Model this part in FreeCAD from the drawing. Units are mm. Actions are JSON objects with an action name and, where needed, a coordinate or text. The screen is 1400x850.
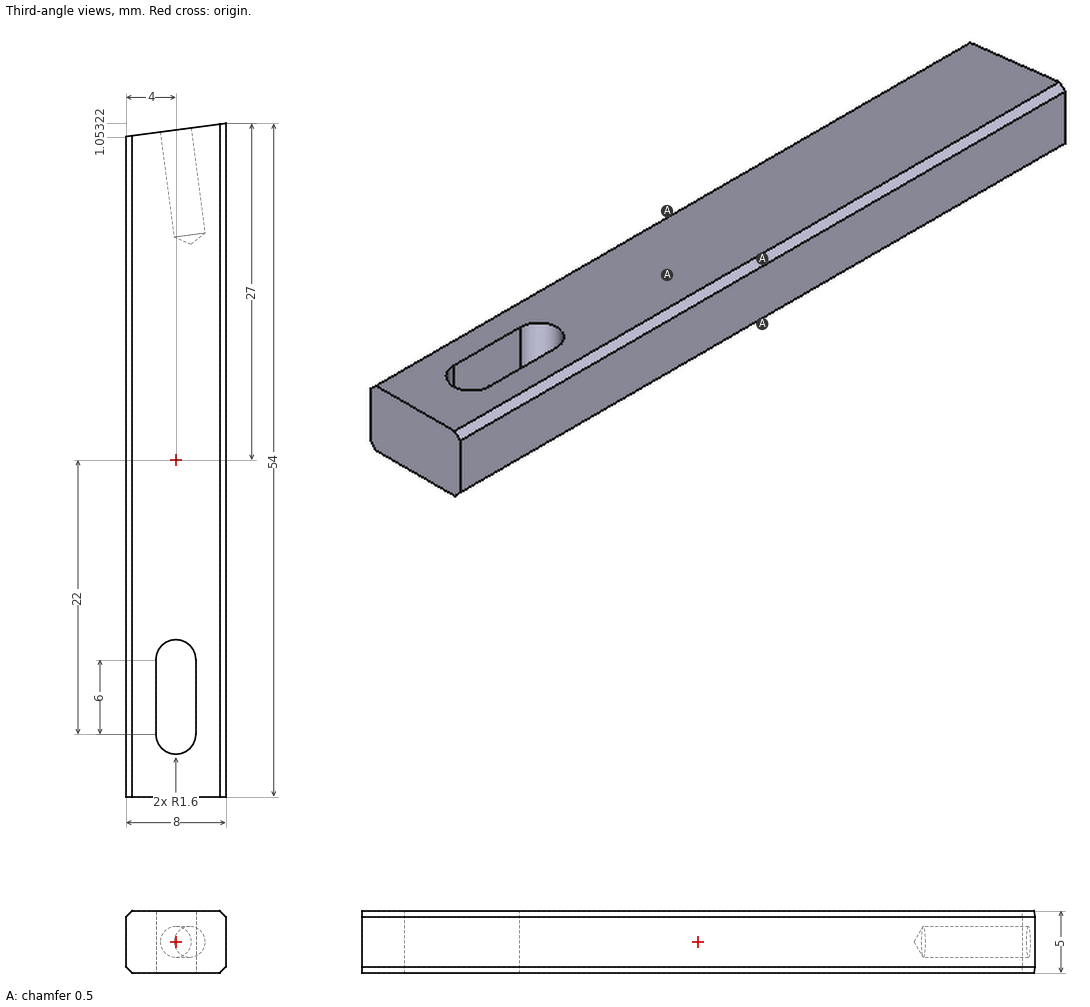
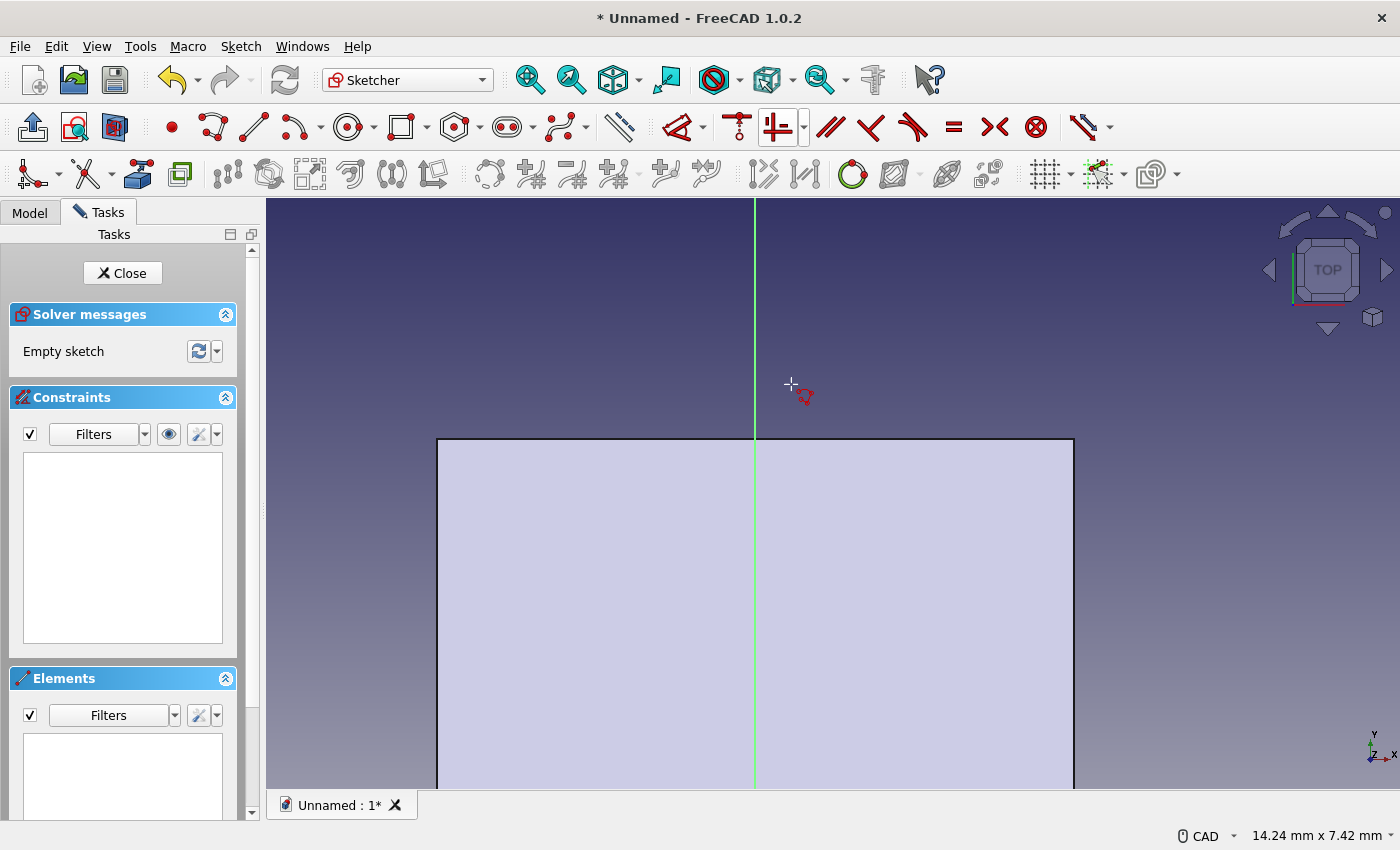
{"action": "left_click", "coordinate": [437, 523]}
{"action": "left_click", "coordinate": [1074, 439]}
{"action": "left_click", "coordinate": [437, 439]}
{"action": "left_click", "coordinate": [437, 524]}
{"action": "key", "text": "Escape"}
{"action": "key", "text": "Escape"}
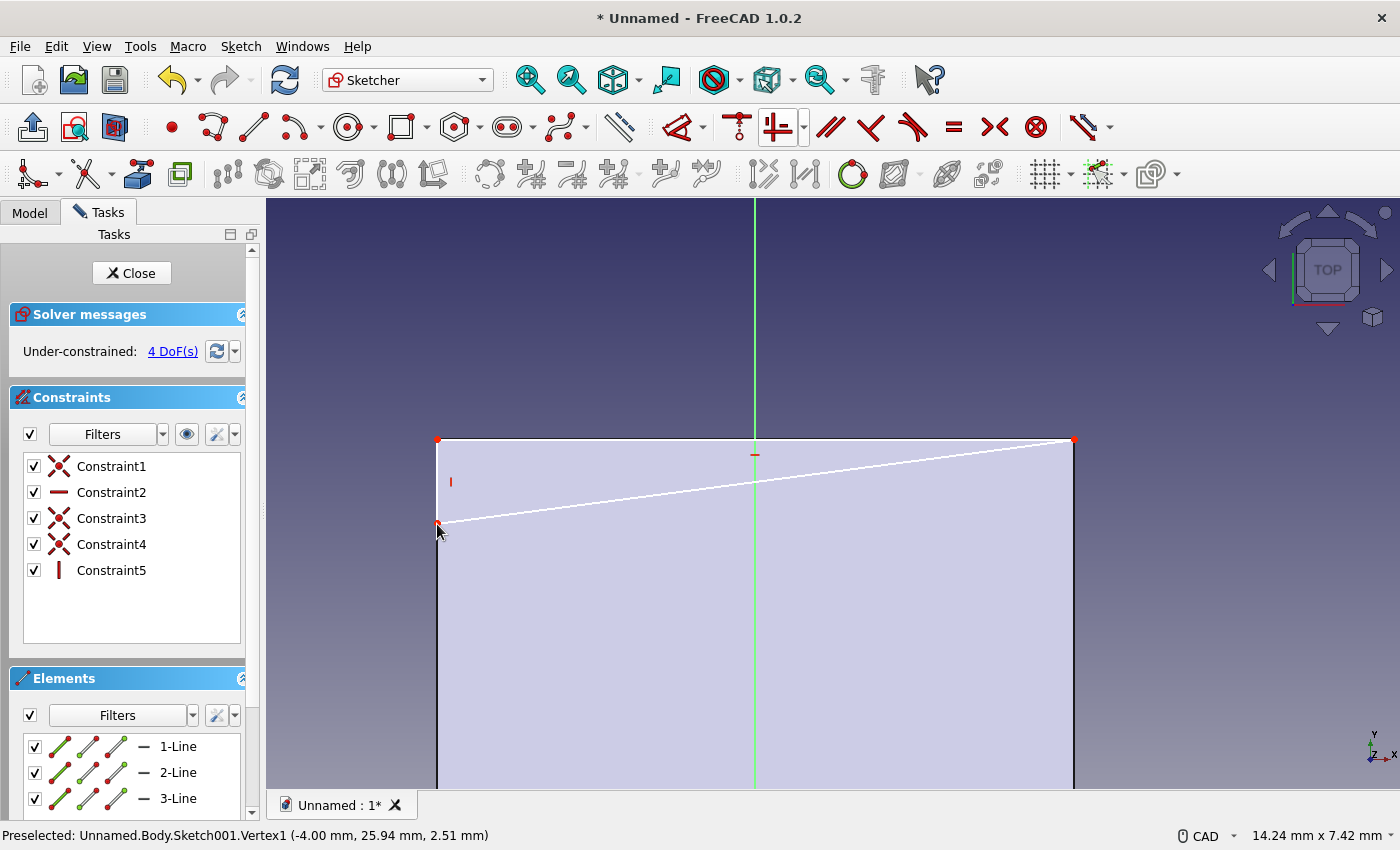
{"action": "left_click", "coordinate": [883, 440]}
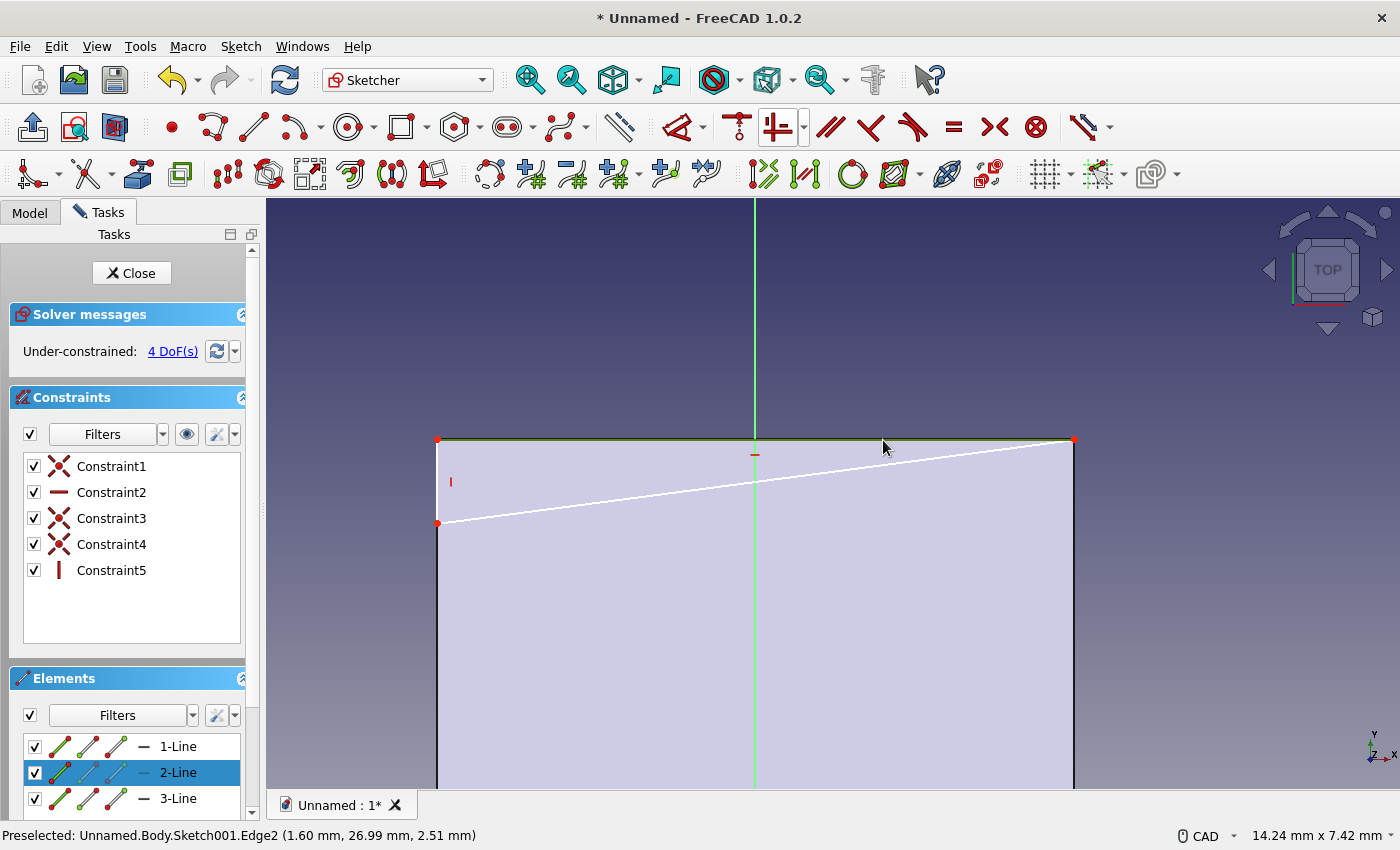
{"action": "key", "text": "l"}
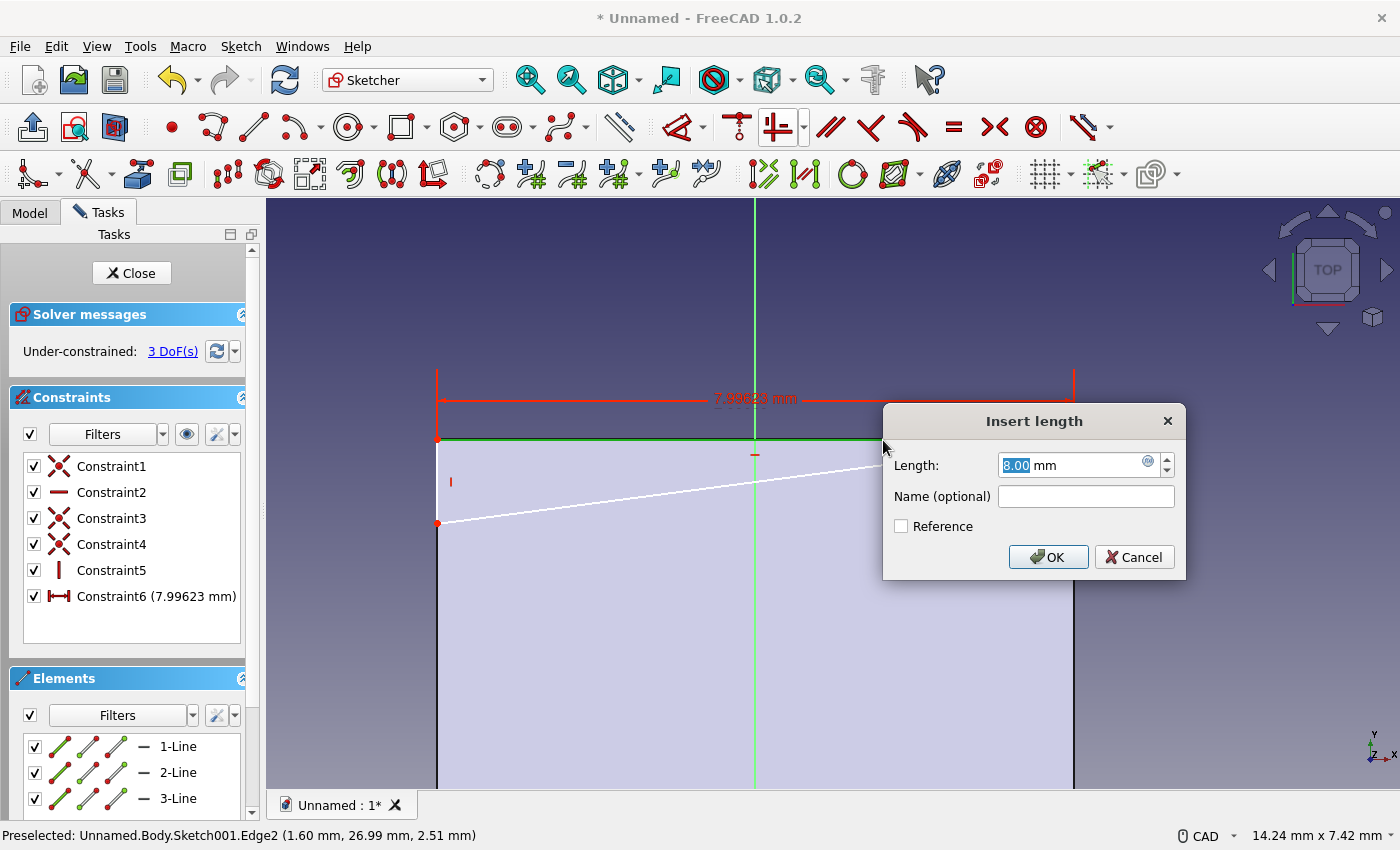
{"action": "type", "text": "8"}
{"action": "key", "text": "Return"}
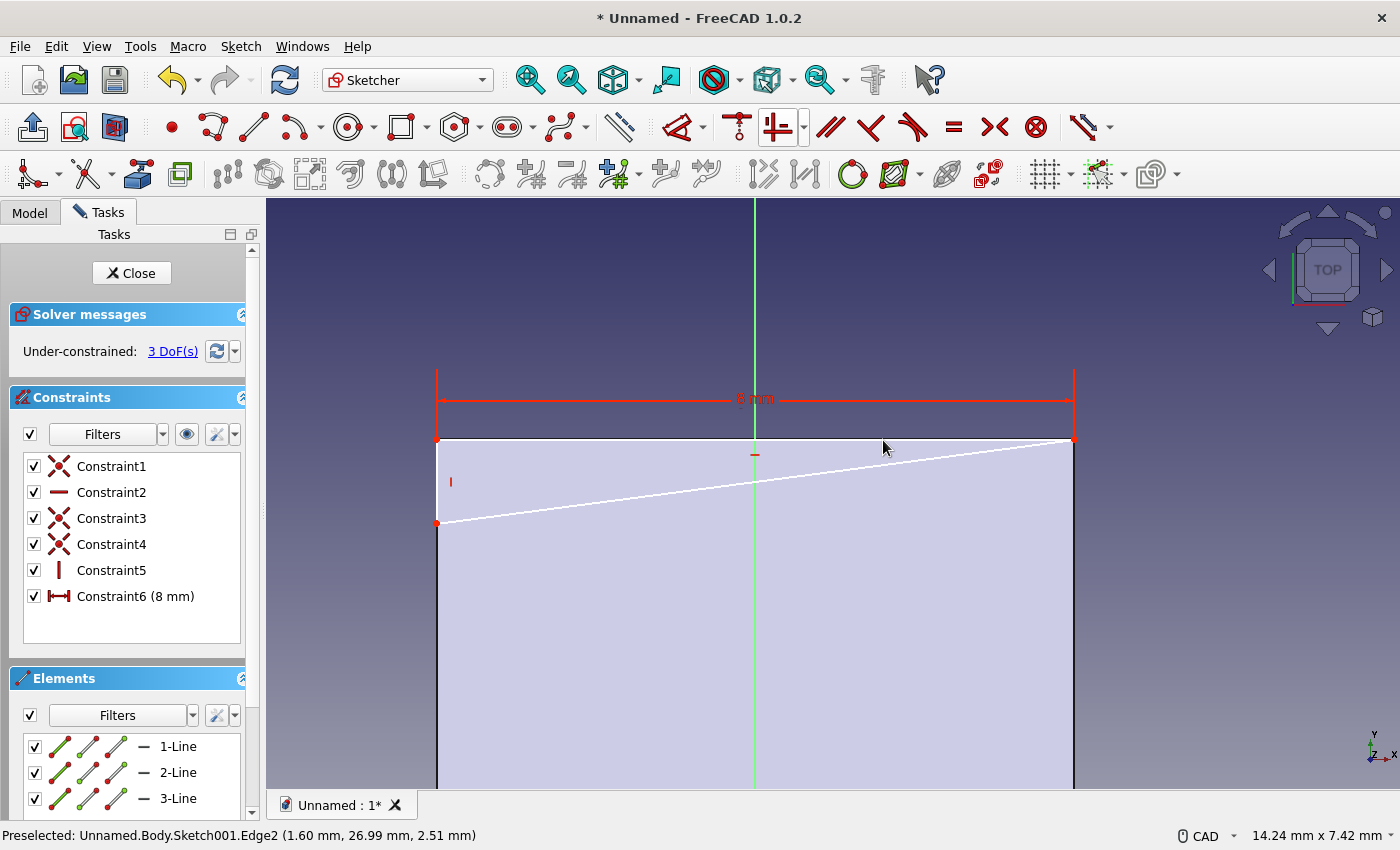
{"action": "left_click", "coordinate": [437, 524]}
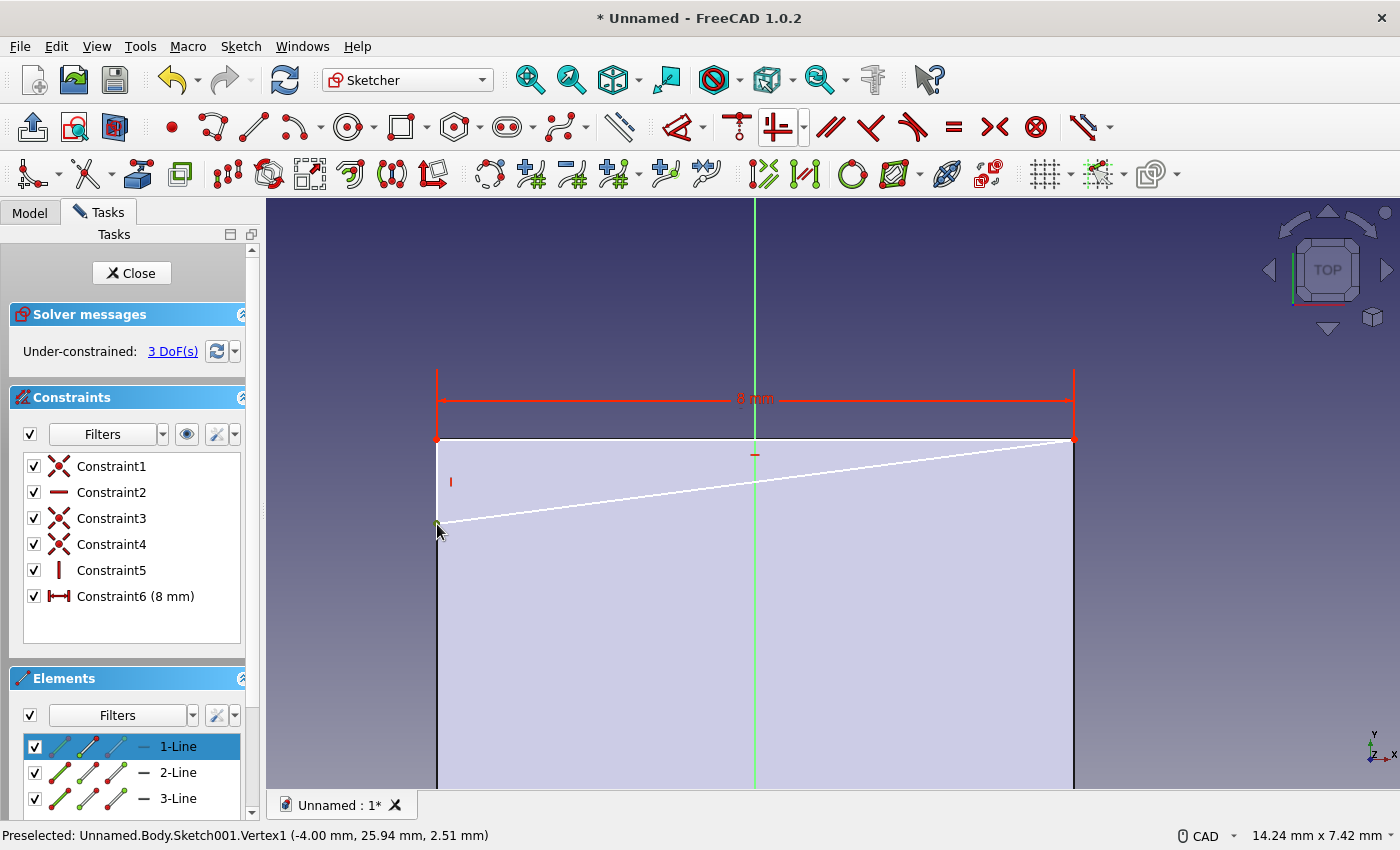
{"action": "key", "text": "l"}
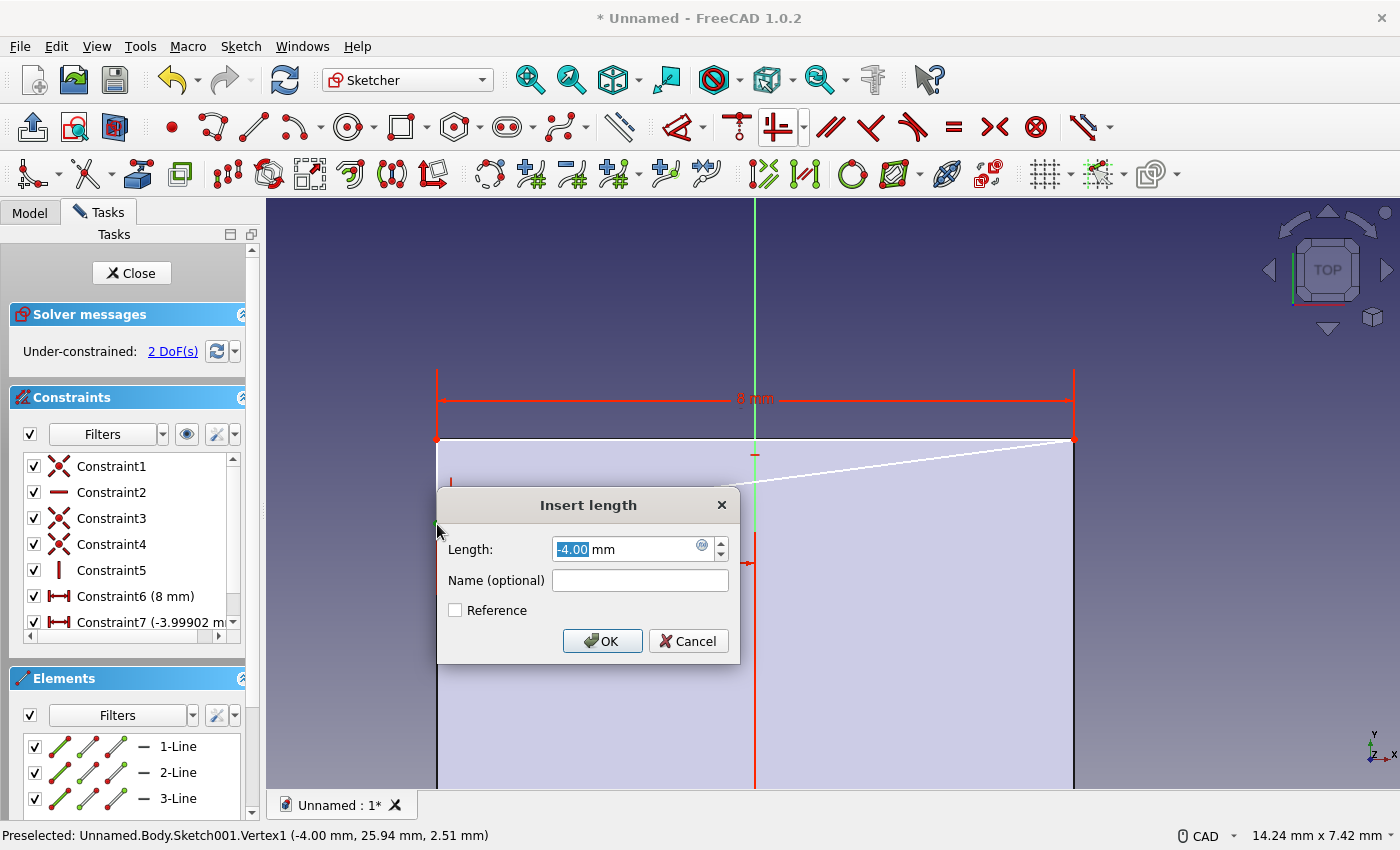
{"action": "type", "text": "-4"}
{"action": "key", "text": "Return"}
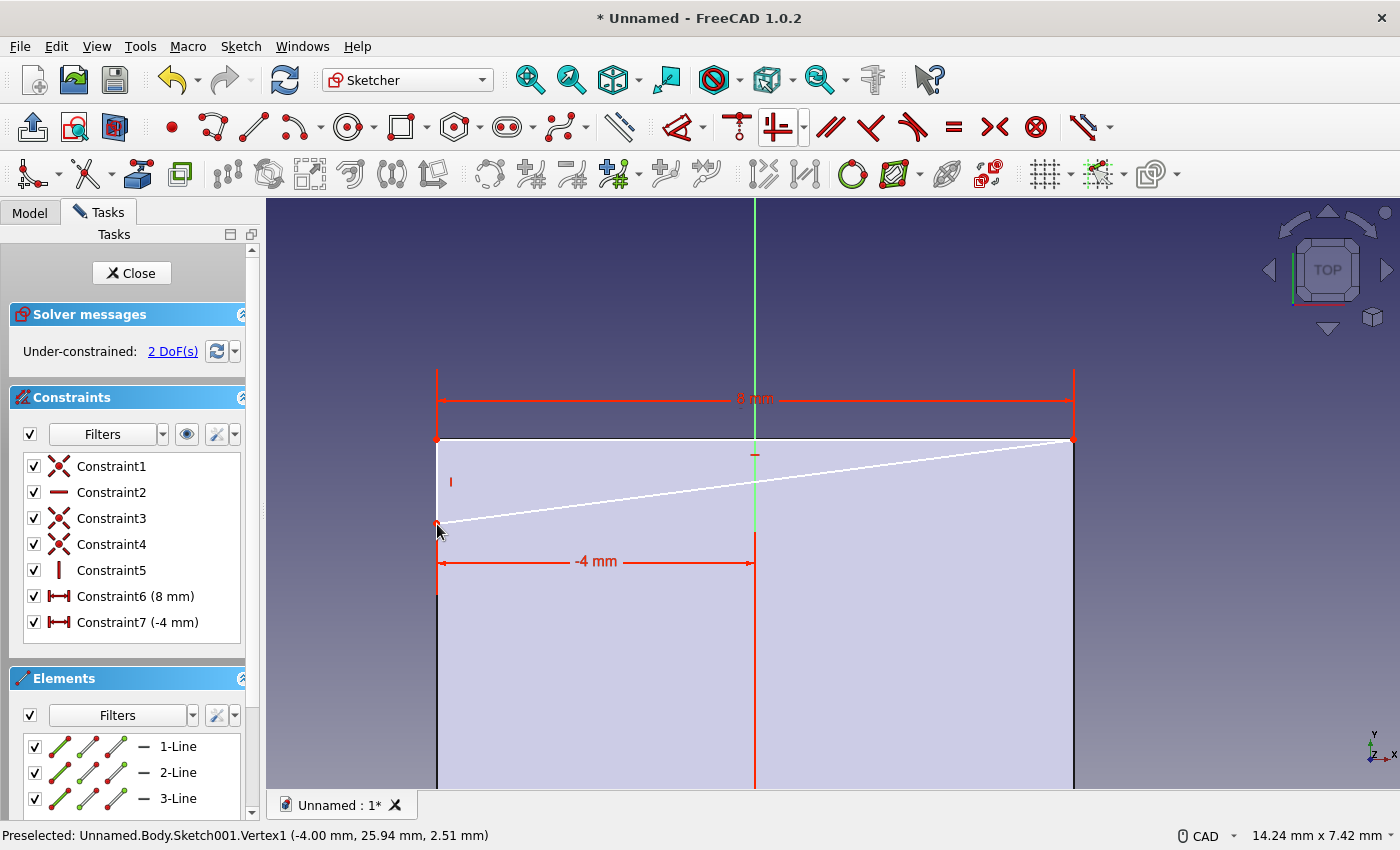
{"action": "left_click", "coordinate": [1074, 440]}